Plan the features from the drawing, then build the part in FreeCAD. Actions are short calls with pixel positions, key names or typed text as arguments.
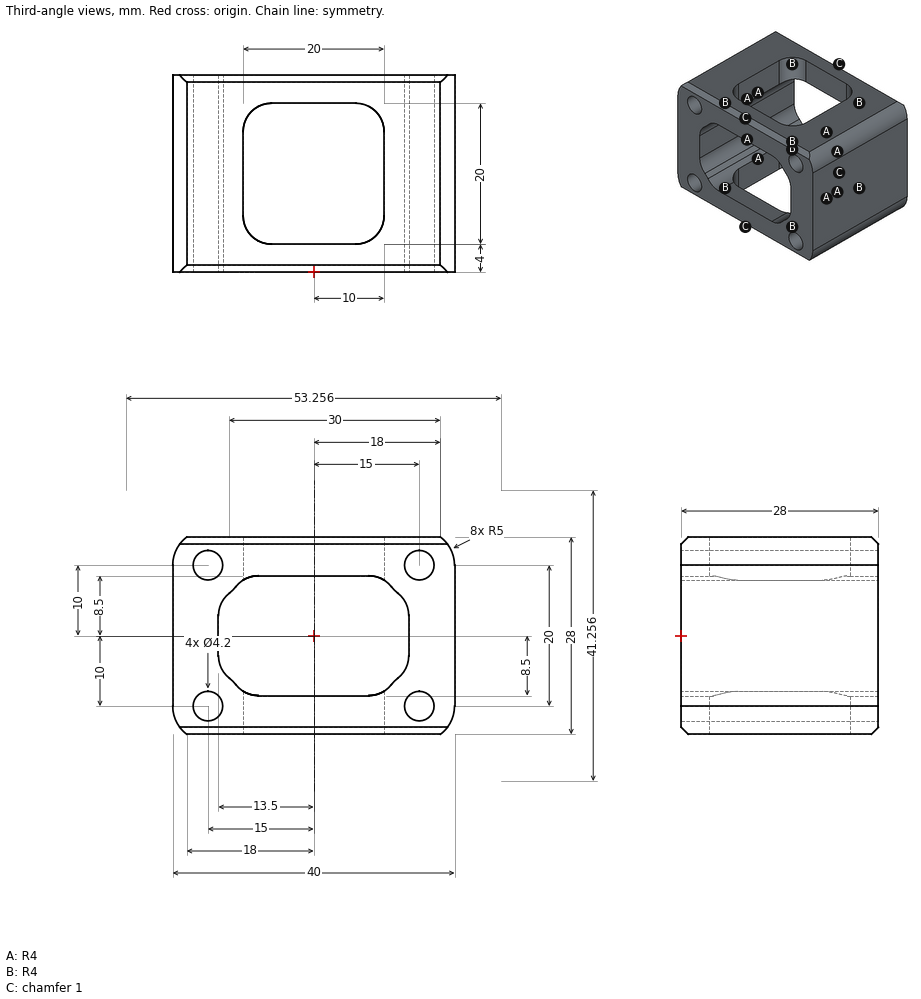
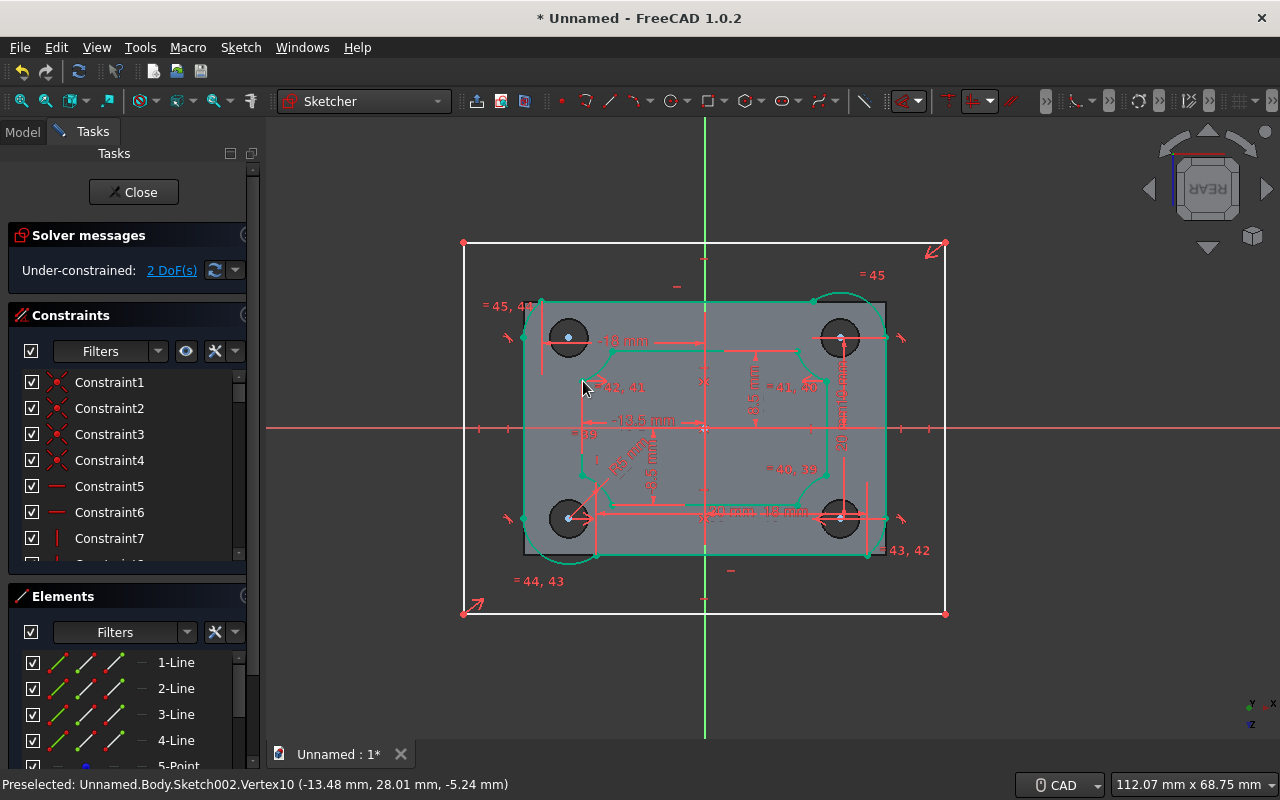
click(608, 614)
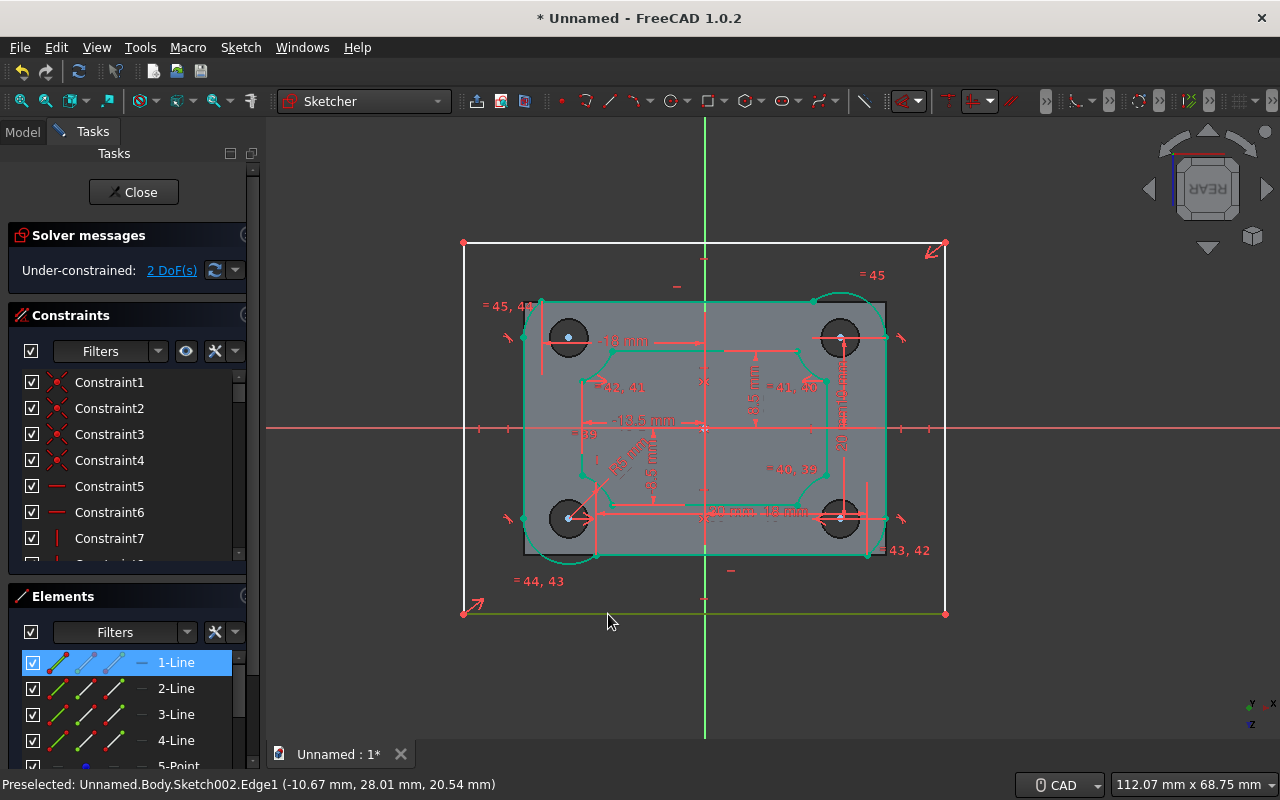
key(l)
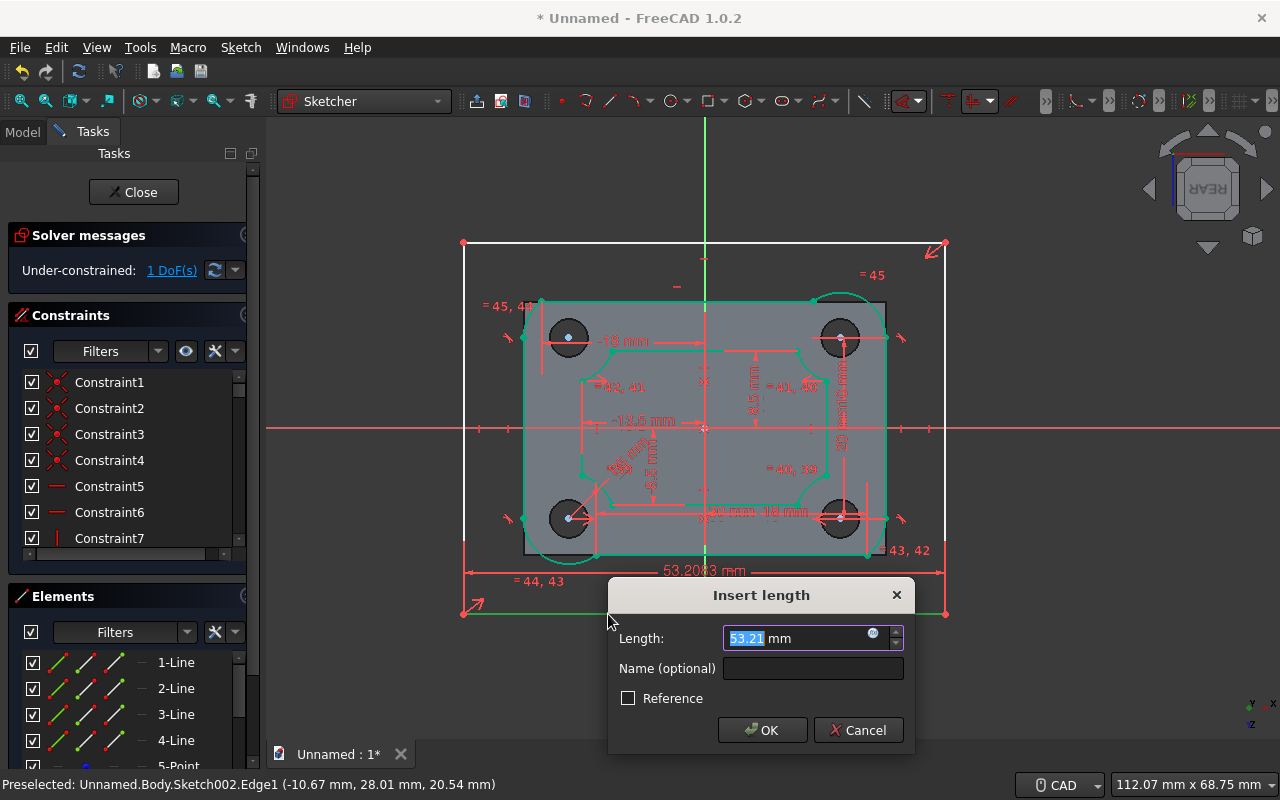
text(53.256)
key(Return)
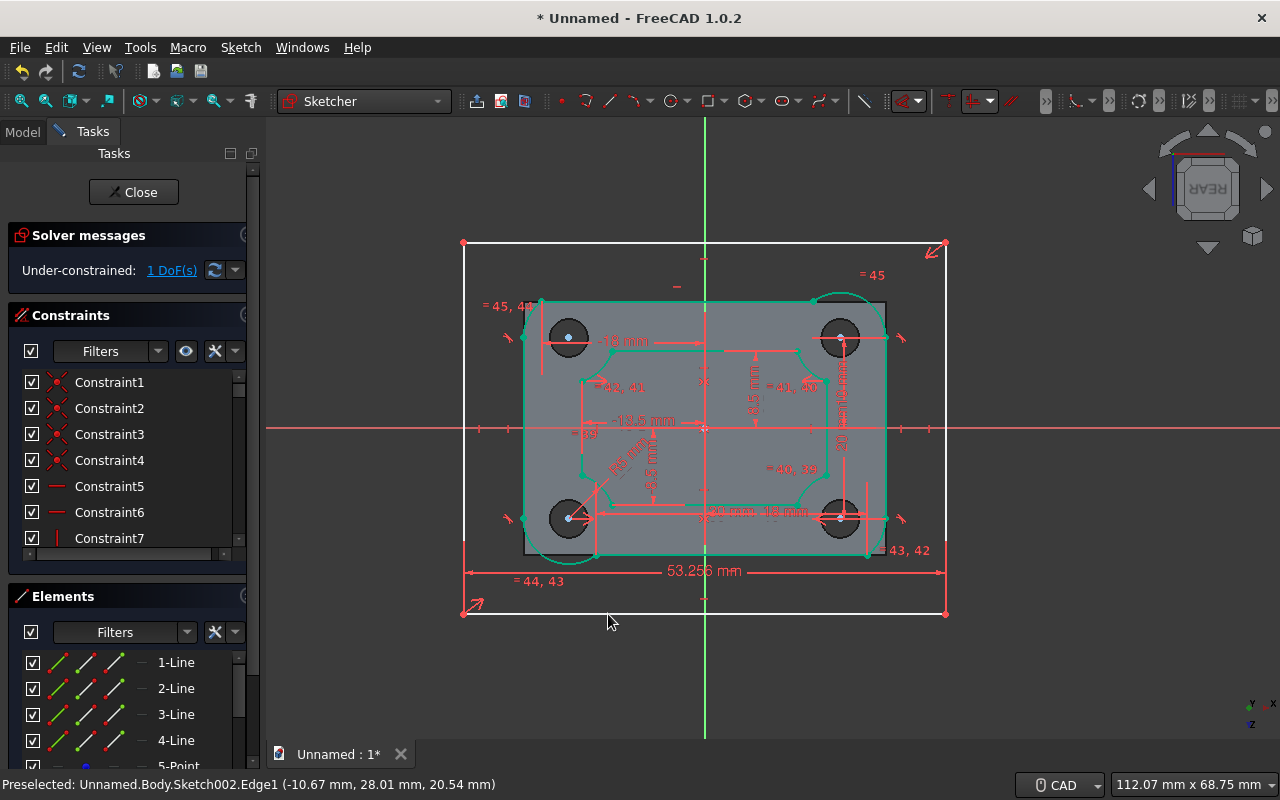
click(946, 503)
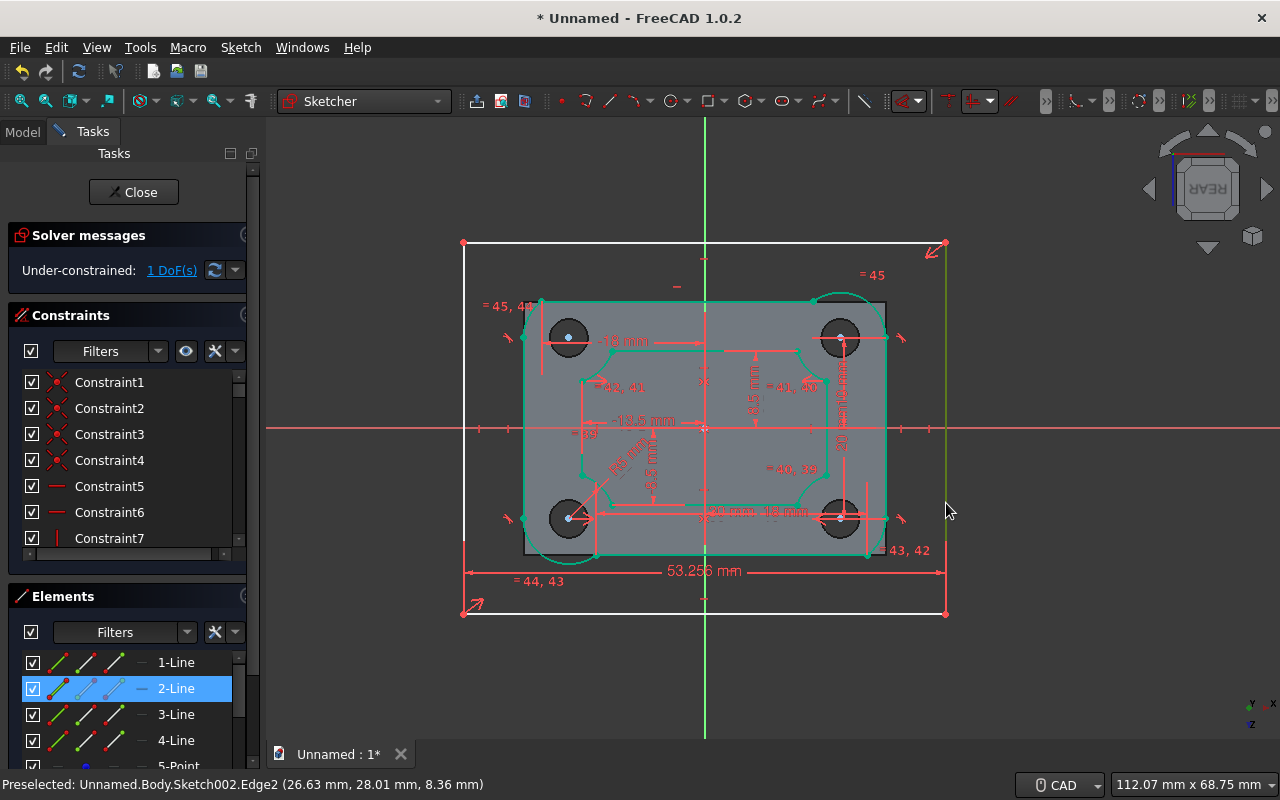
key(i)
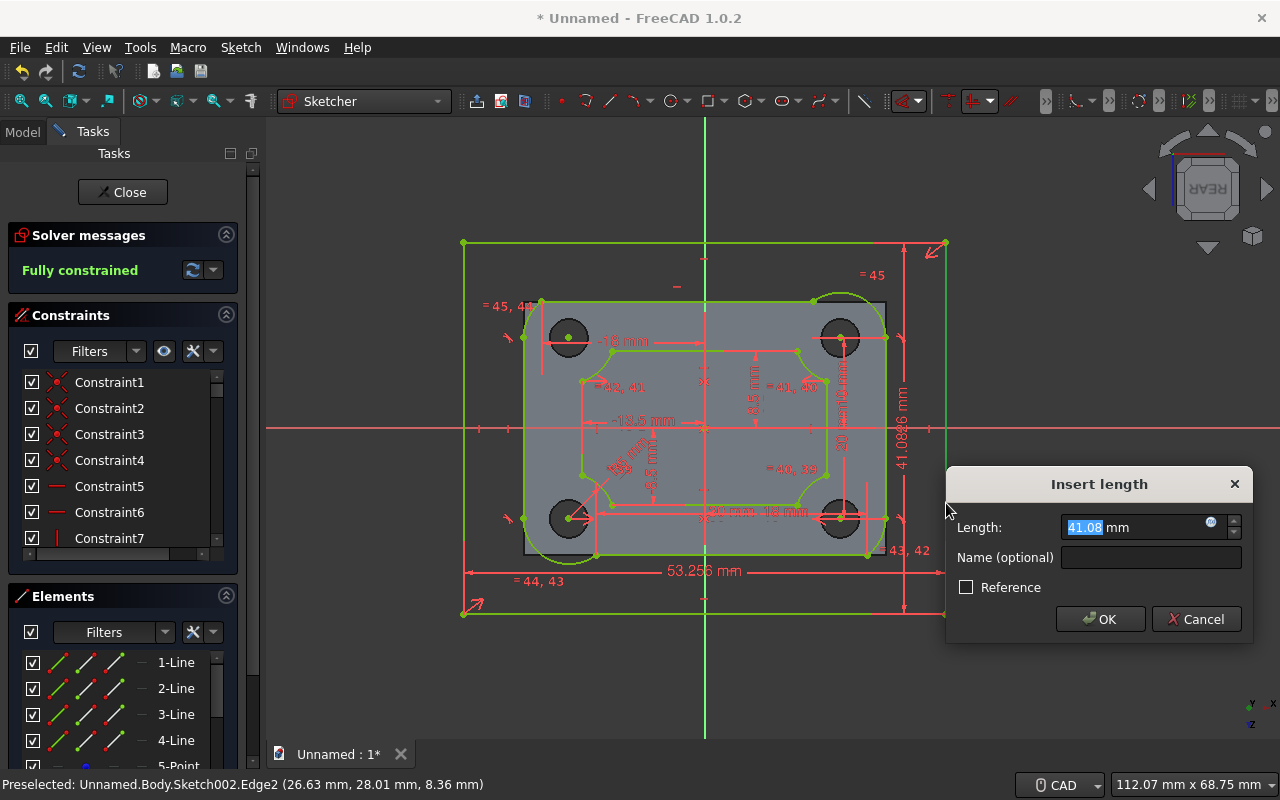
text(41.256)
key(Return)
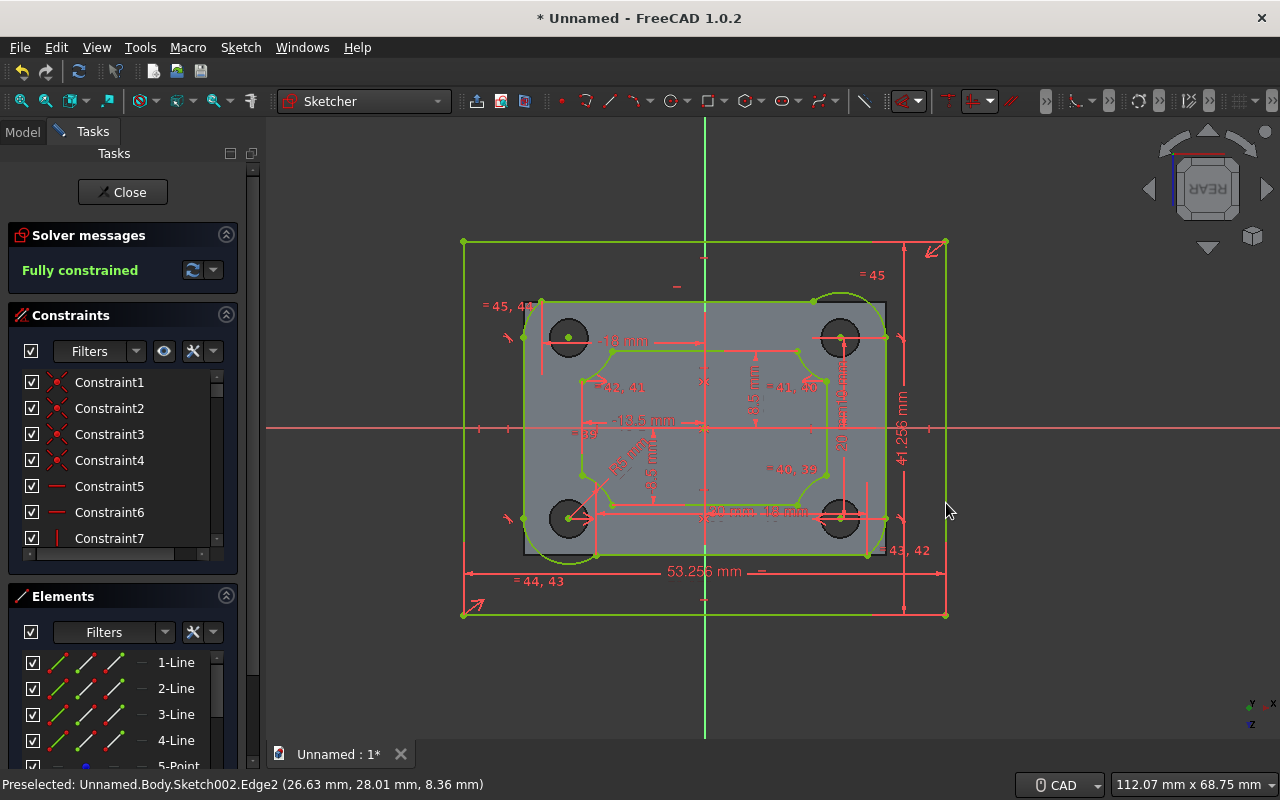
click(123, 192)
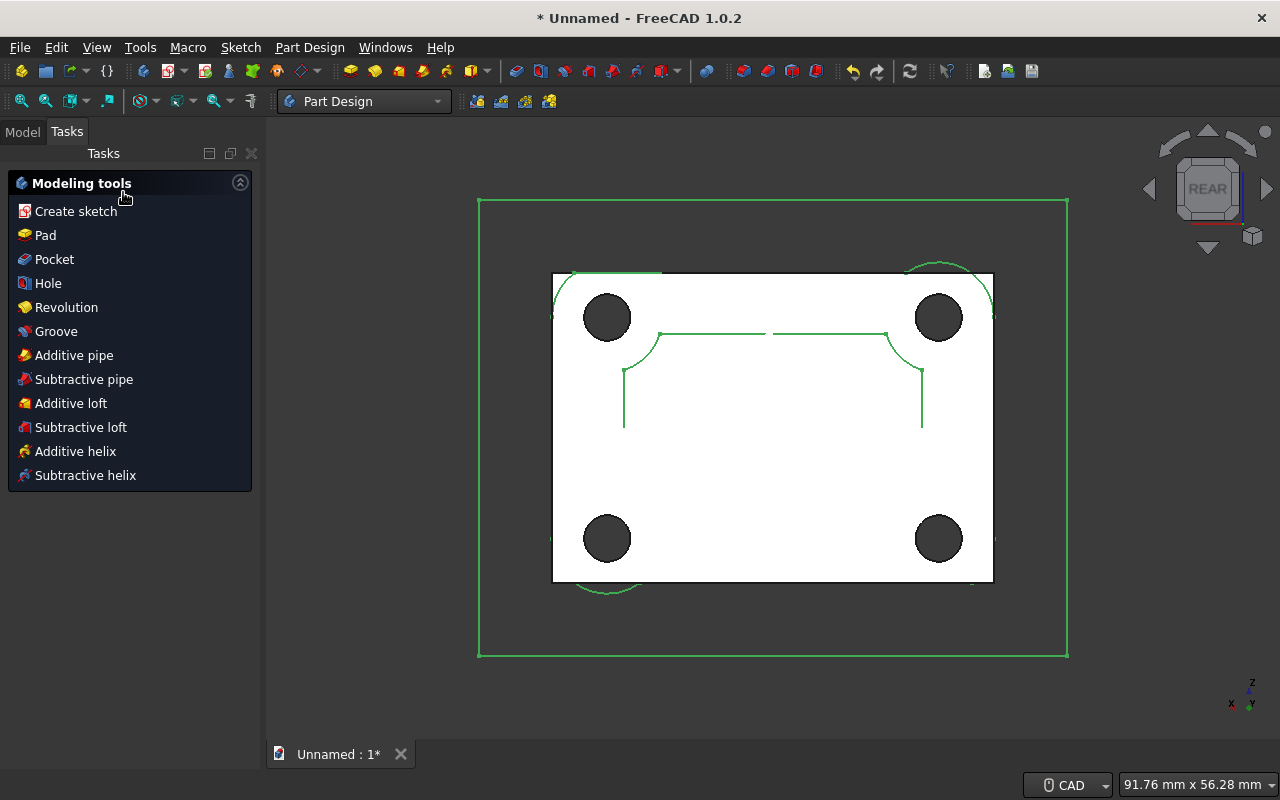
click(518, 72)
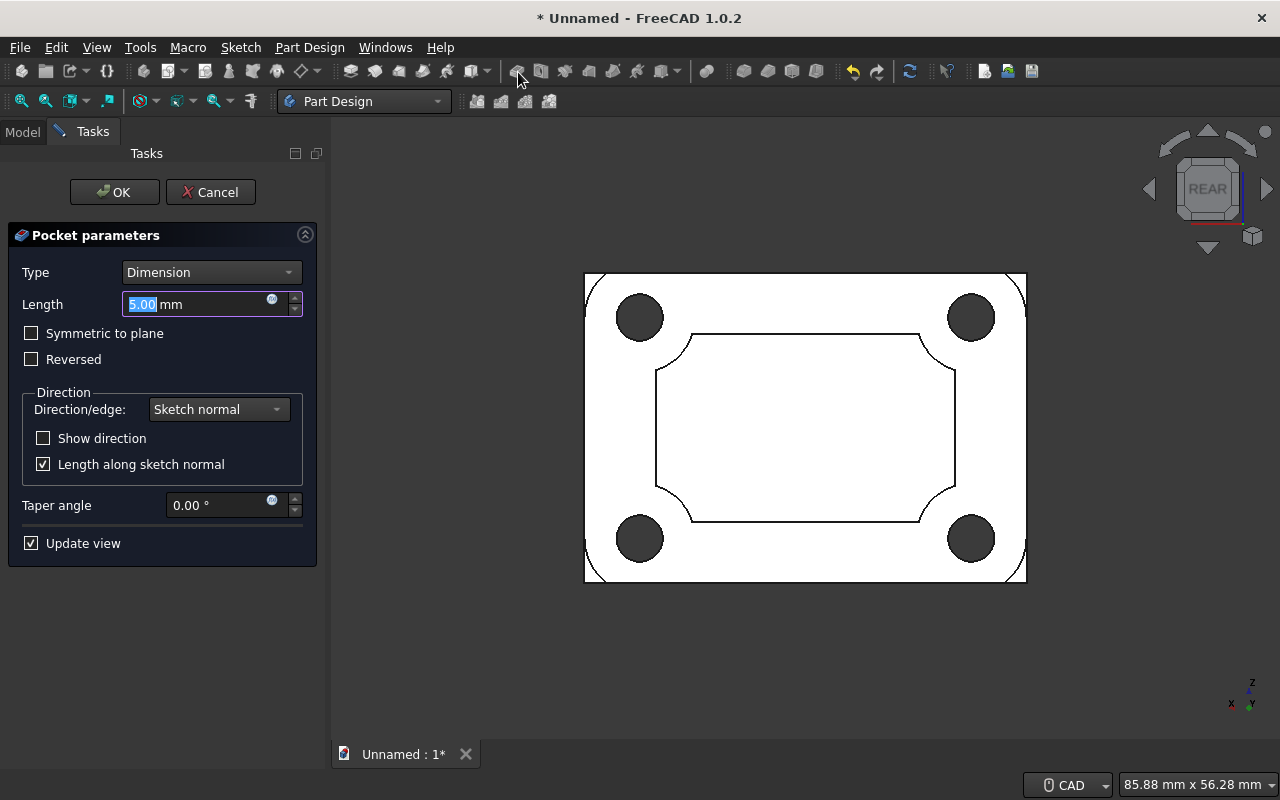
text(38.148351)
key(Tab)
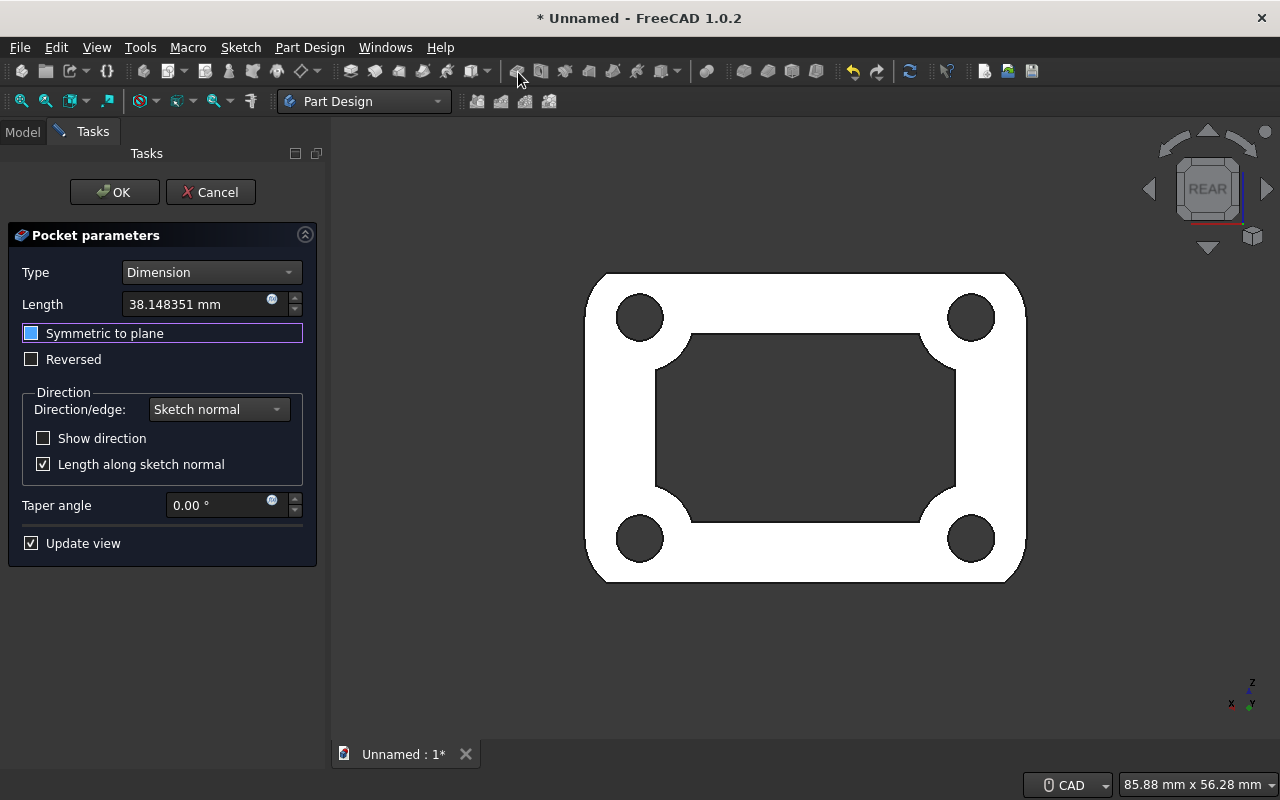
click(115, 192)